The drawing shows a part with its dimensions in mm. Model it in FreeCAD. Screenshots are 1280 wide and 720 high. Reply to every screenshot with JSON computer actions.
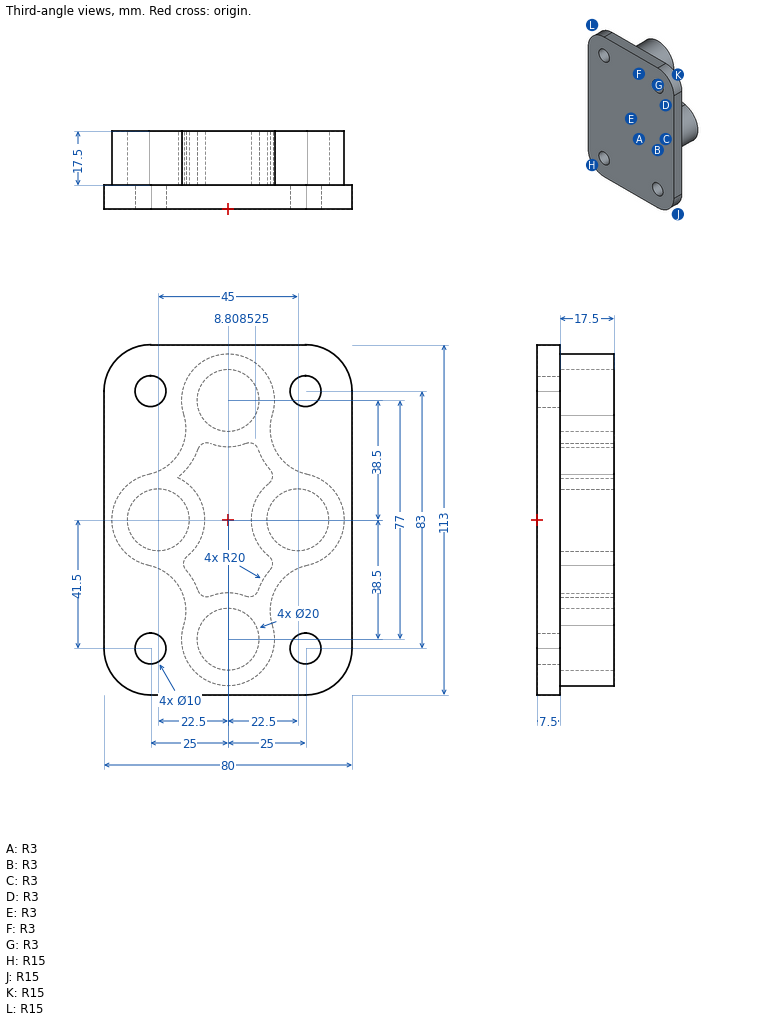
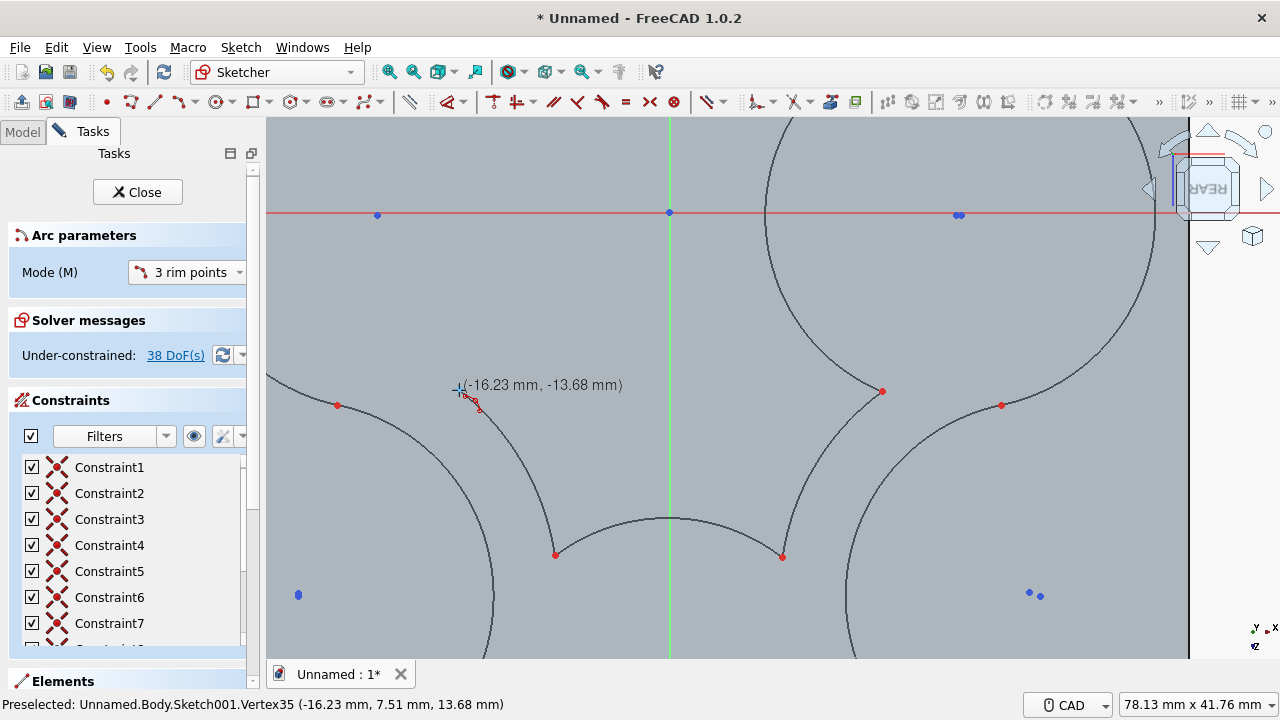
{"action": "scroll", "coordinate": [716, 445], "scroll_direction": "down", "scroll_amount": 7}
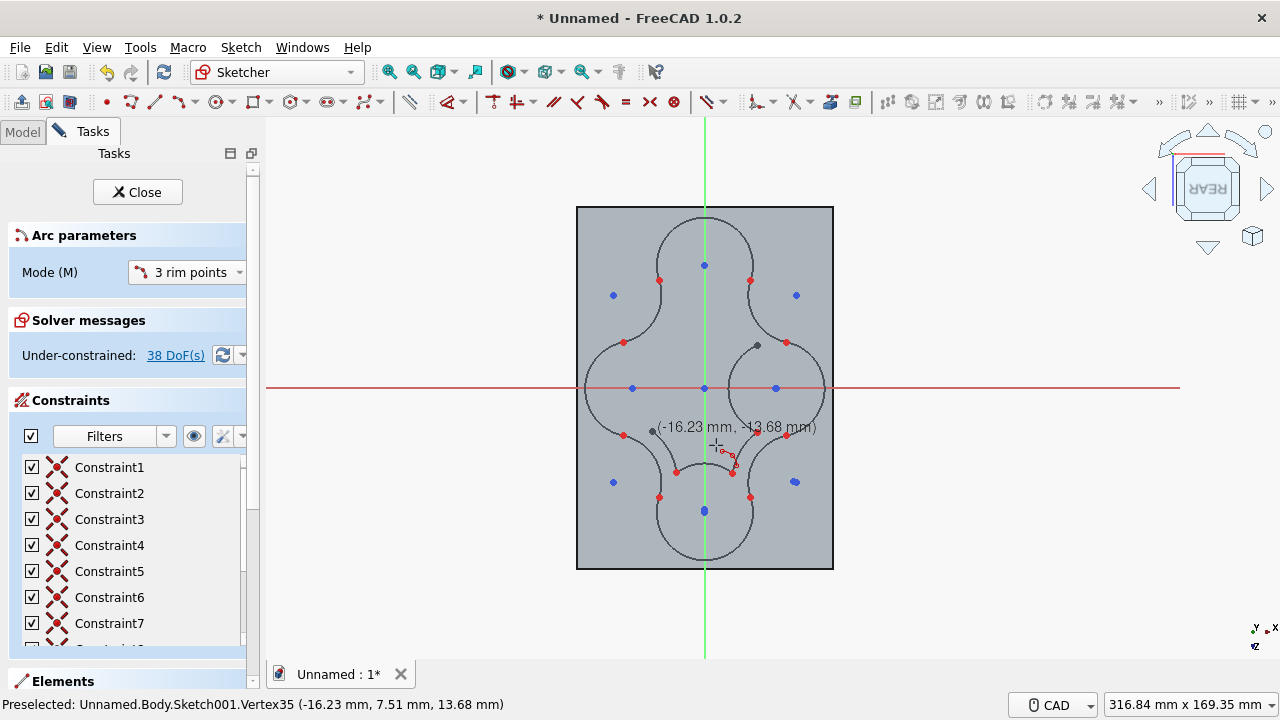
{"action": "left_click", "coordinate": [653, 344]}
{"action": "left_click", "coordinate": [676, 409]}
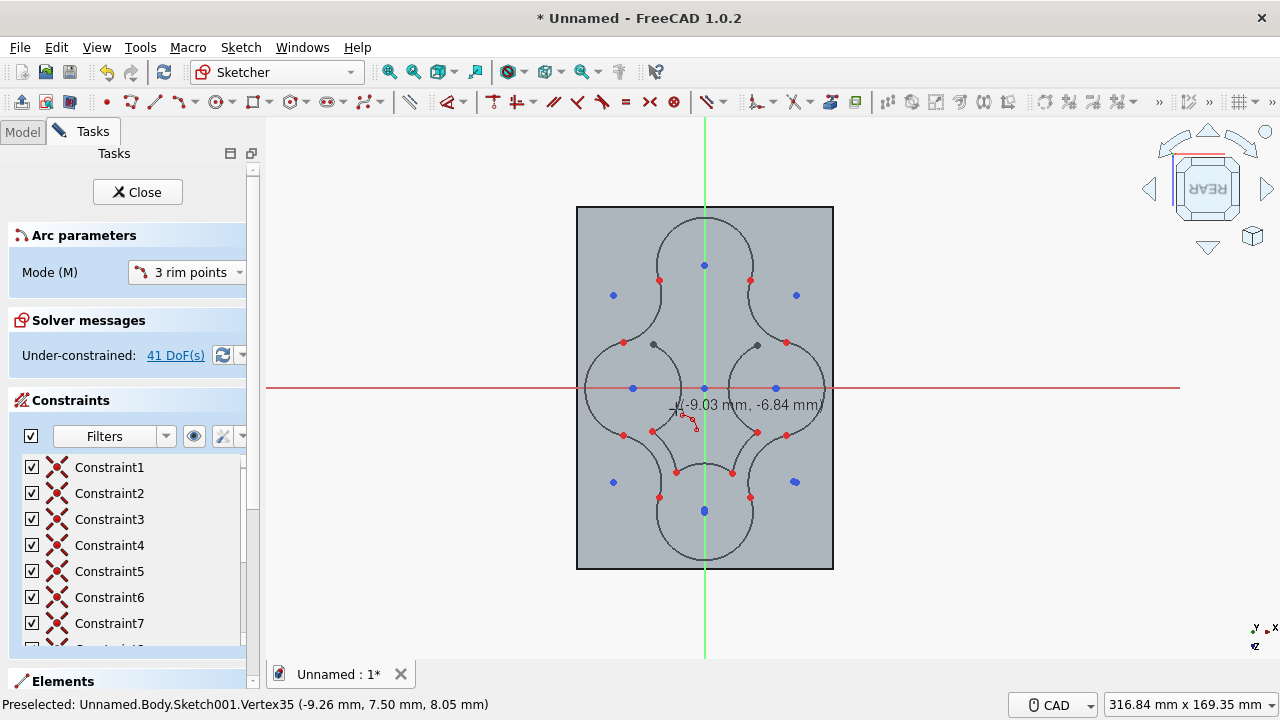
{"action": "left_click", "coordinate": [653, 345]}
{"action": "left_click", "coordinate": [677, 304]}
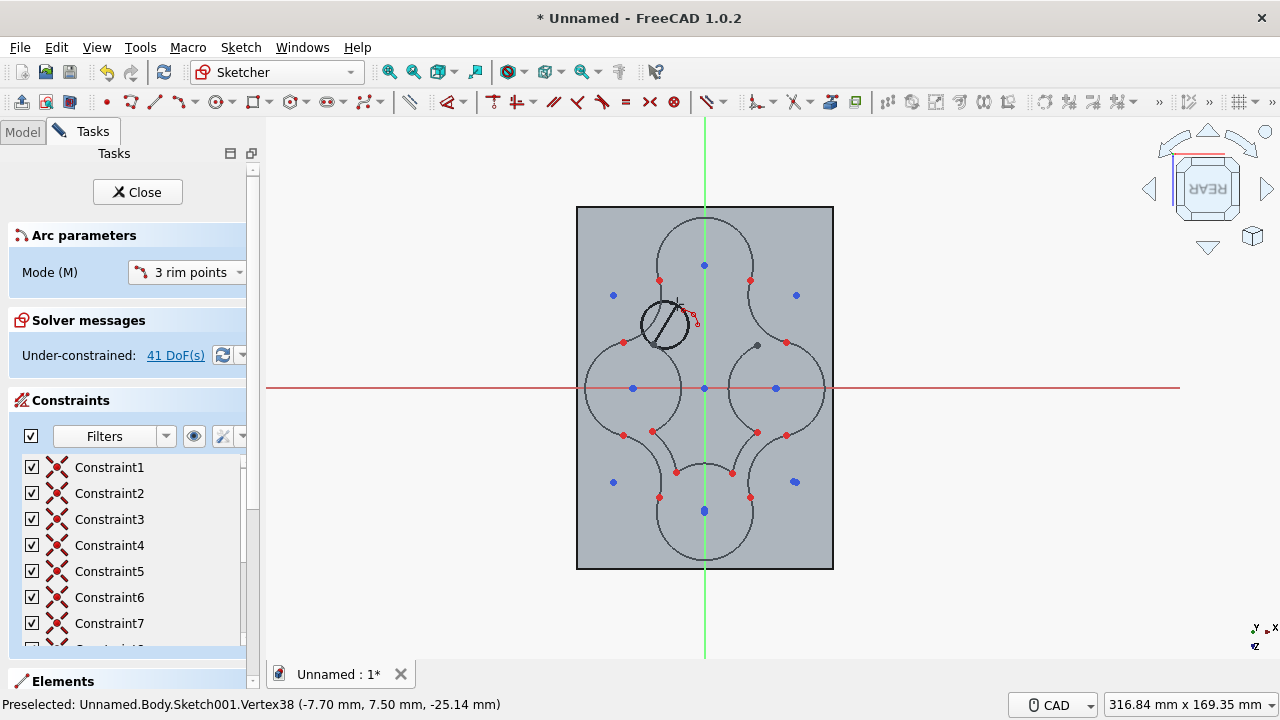
{"action": "scroll", "coordinate": [669, 326], "scroll_direction": "up", "scroll_amount": 7}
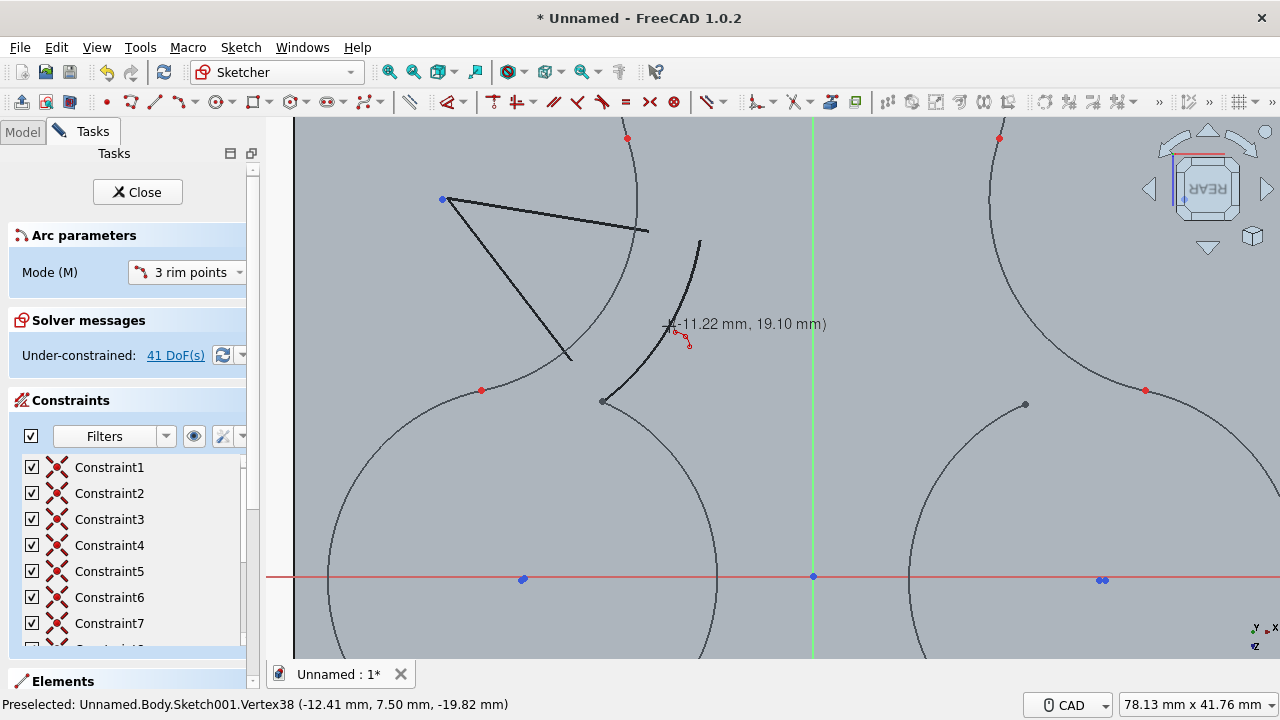
{"action": "left_click", "coordinate": [667, 326]}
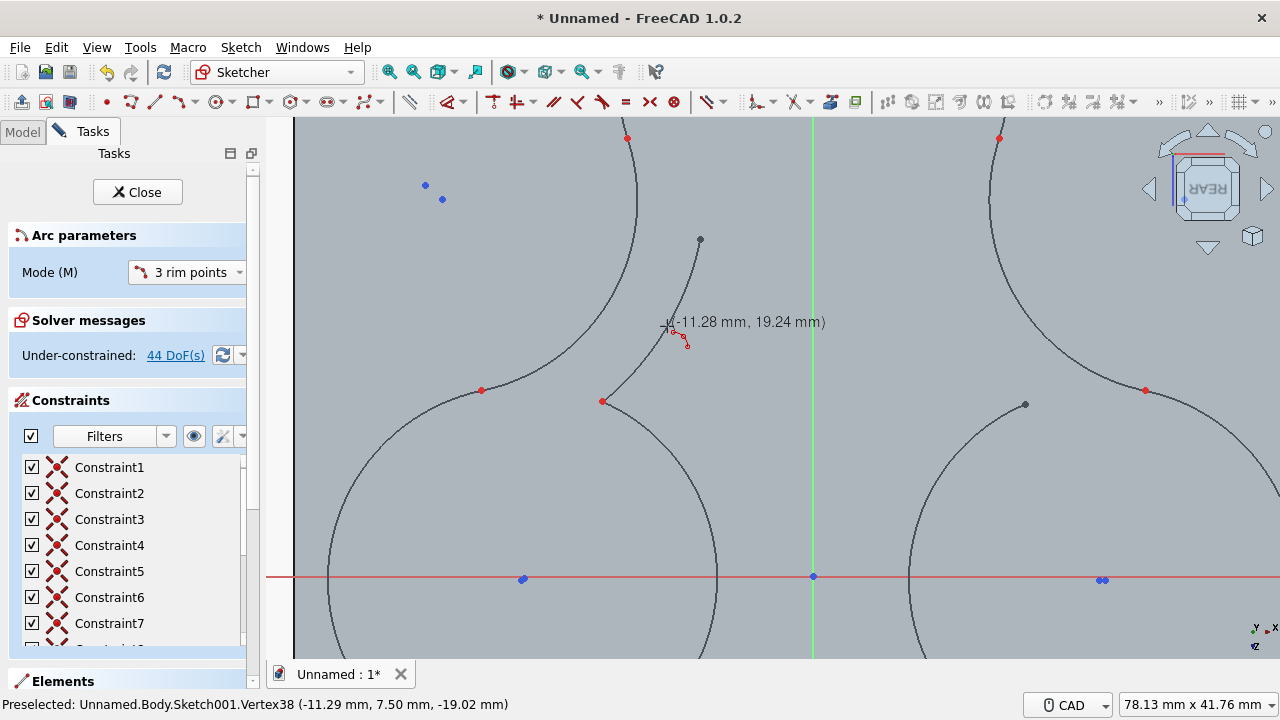
{"action": "left_click", "coordinate": [700, 240]}
{"action": "left_click", "coordinate": [928, 235]}
{"action": "left_click", "coordinate": [765, 266]}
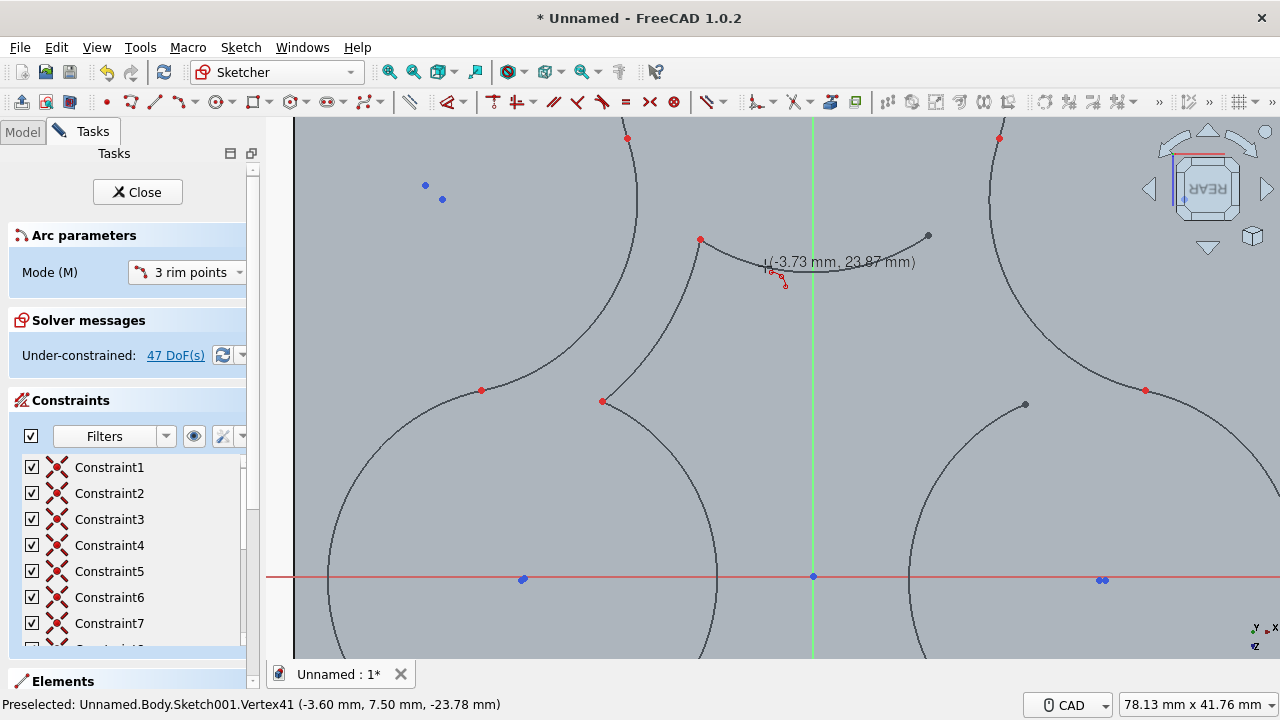
{"action": "left_click", "coordinate": [928, 236]}
{"action": "left_click", "coordinate": [1026, 404]}
{"action": "left_click", "coordinate": [960, 326]}
{"action": "key", "text": "Escape"}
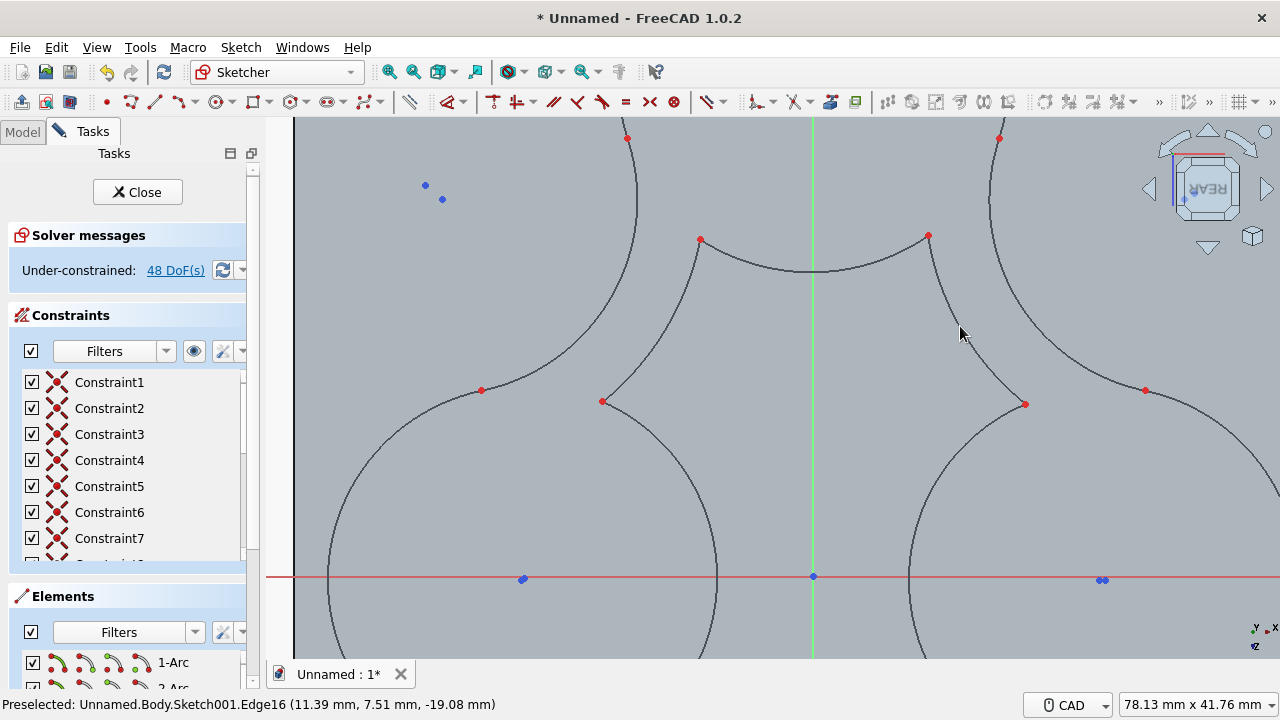
{"action": "left_click", "coordinate": [356, 480]}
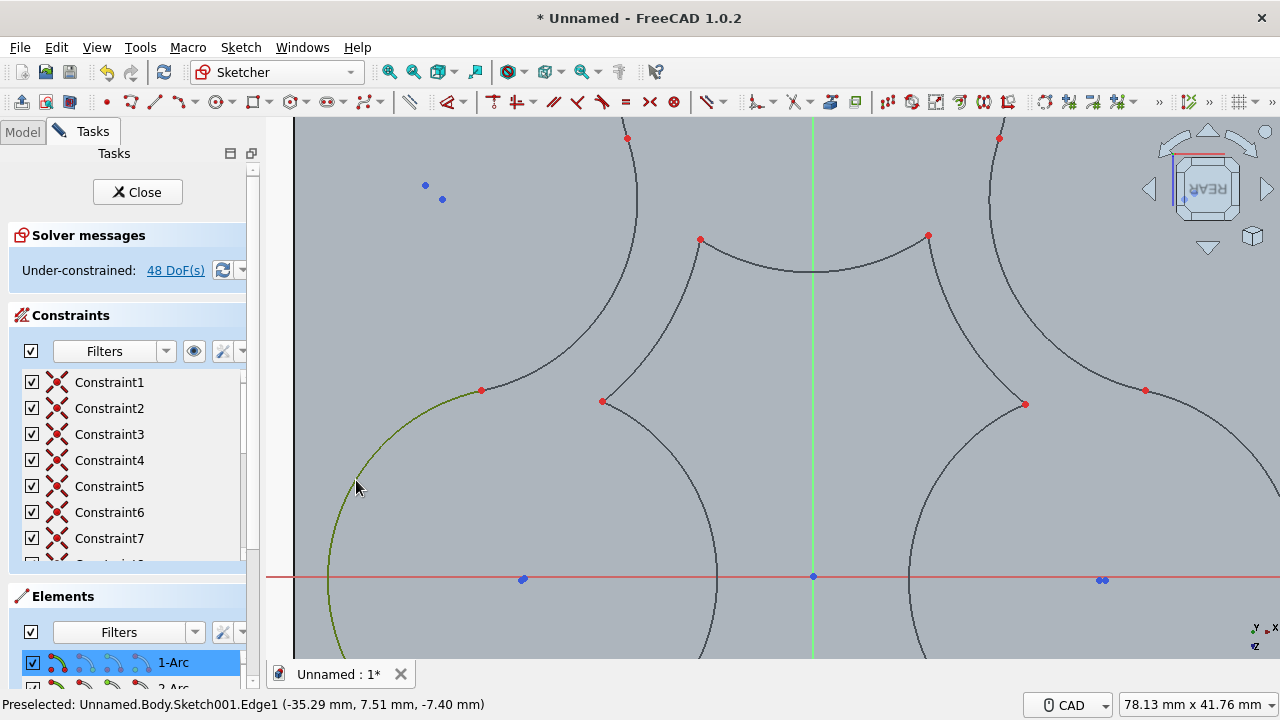
{"action": "scroll", "coordinate": [669, 326], "scroll_direction": "down", "scroll_amount": 7}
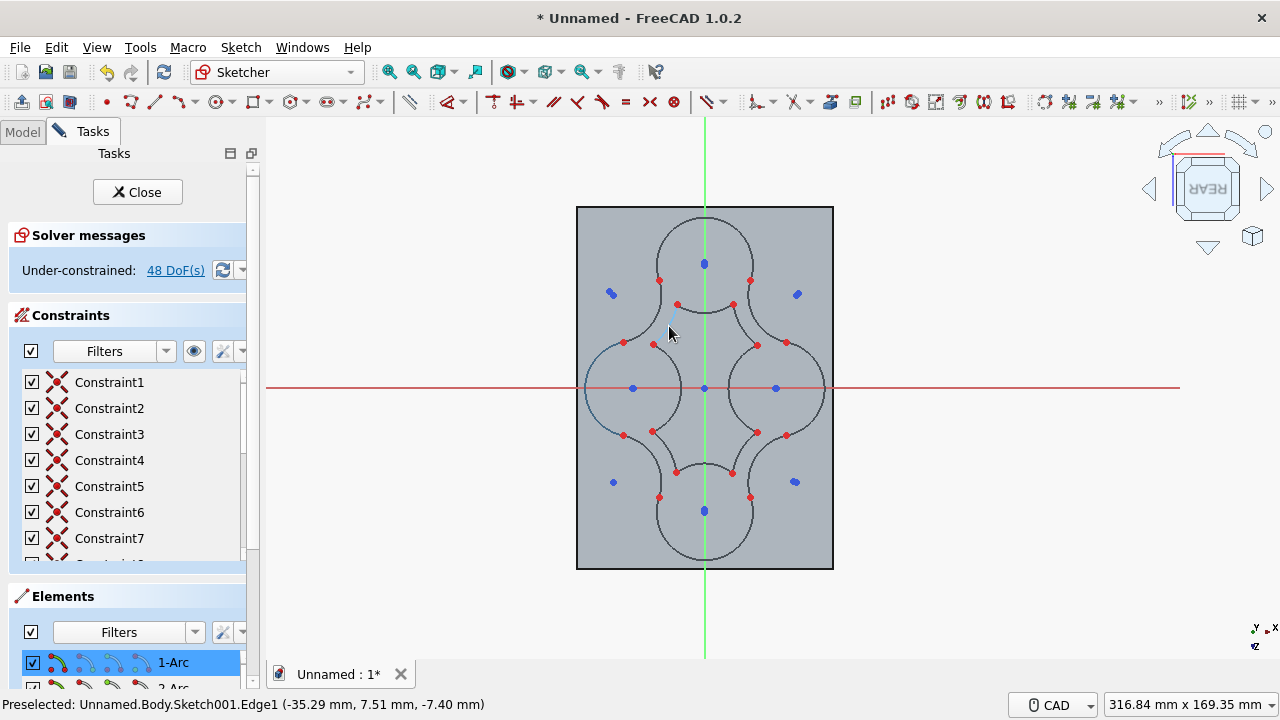
{"action": "left_click", "coordinate": [661, 474]}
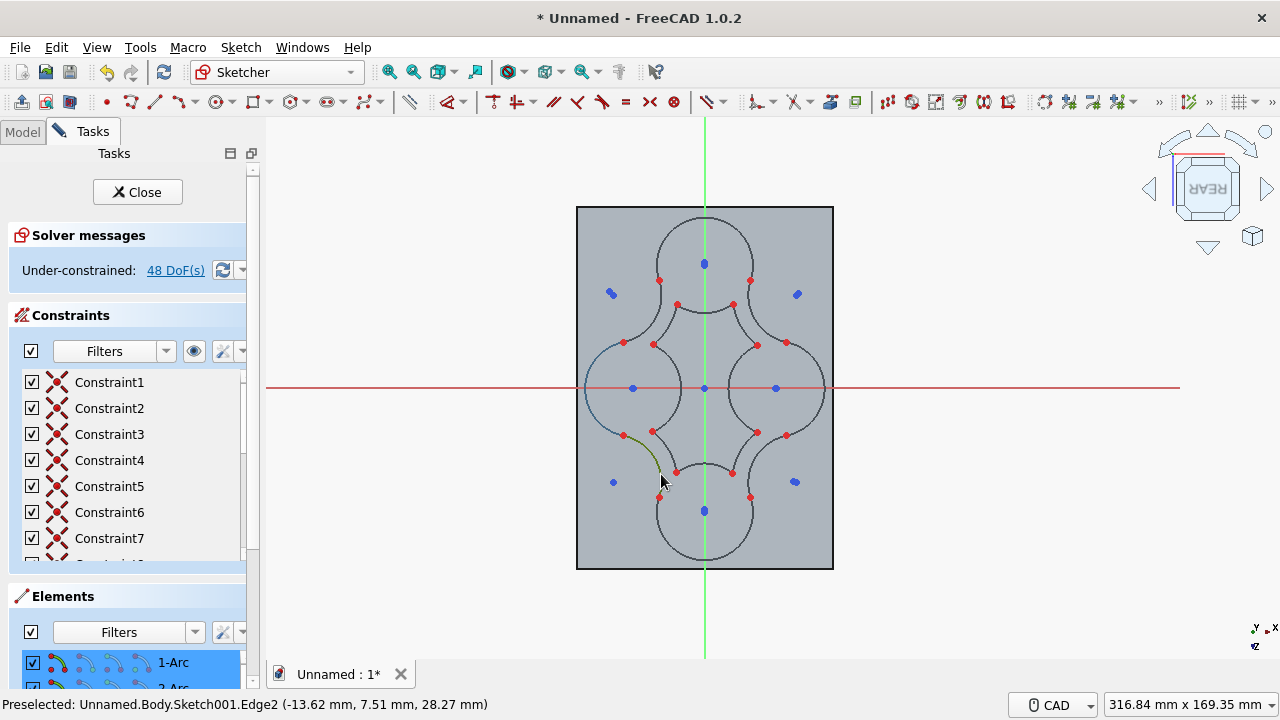
{"action": "left_click", "coordinate": [602, 102]}